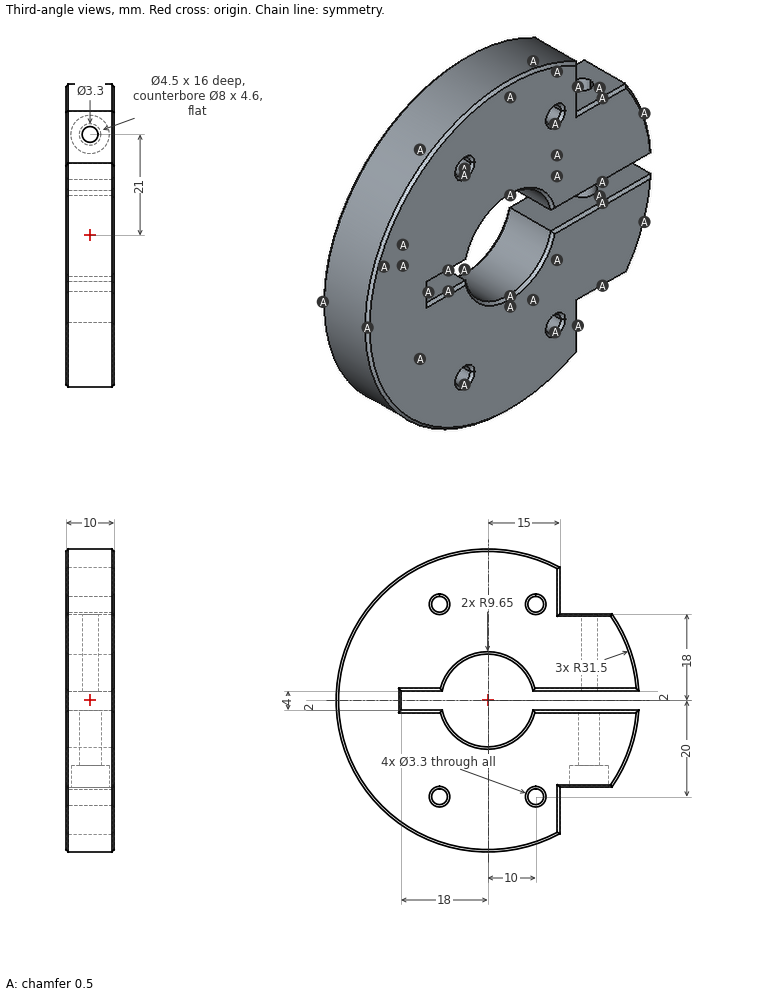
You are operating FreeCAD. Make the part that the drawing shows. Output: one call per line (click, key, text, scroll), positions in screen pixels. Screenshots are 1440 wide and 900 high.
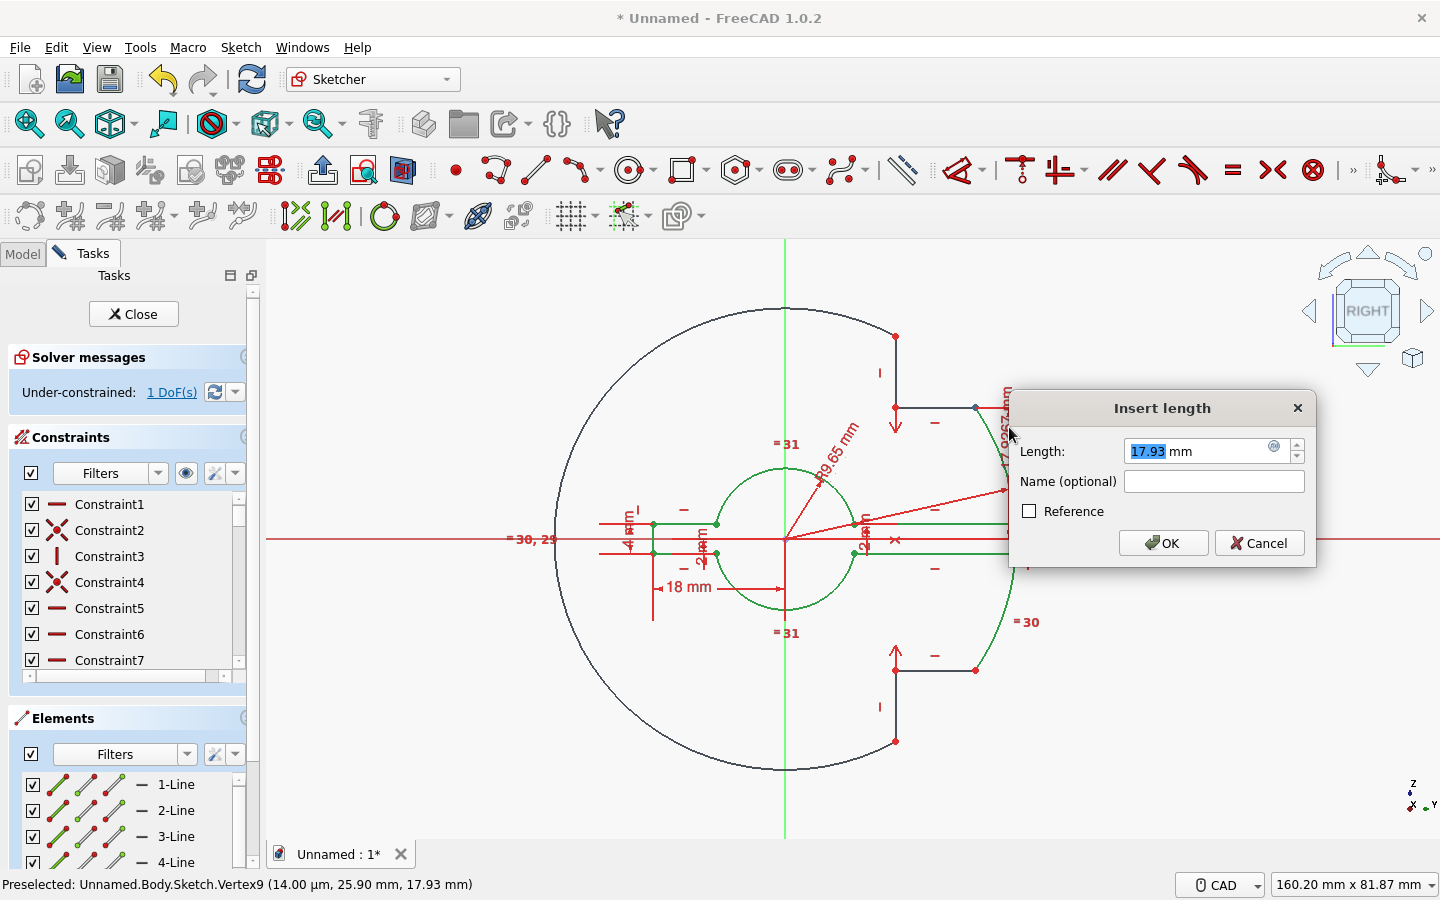
text(18)
key(Return)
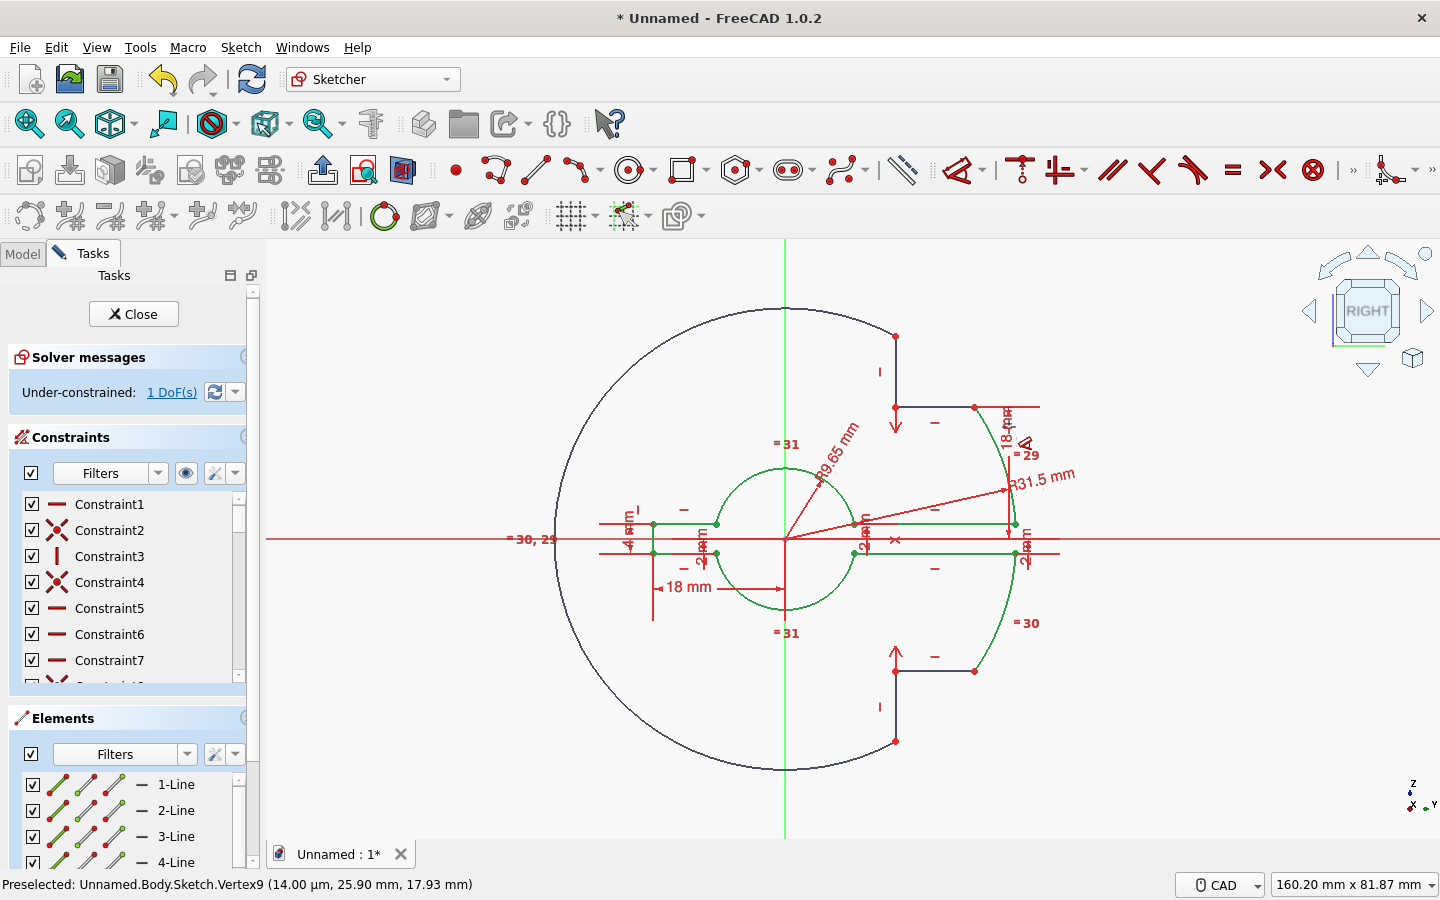
click(896, 407)
click(840, 373)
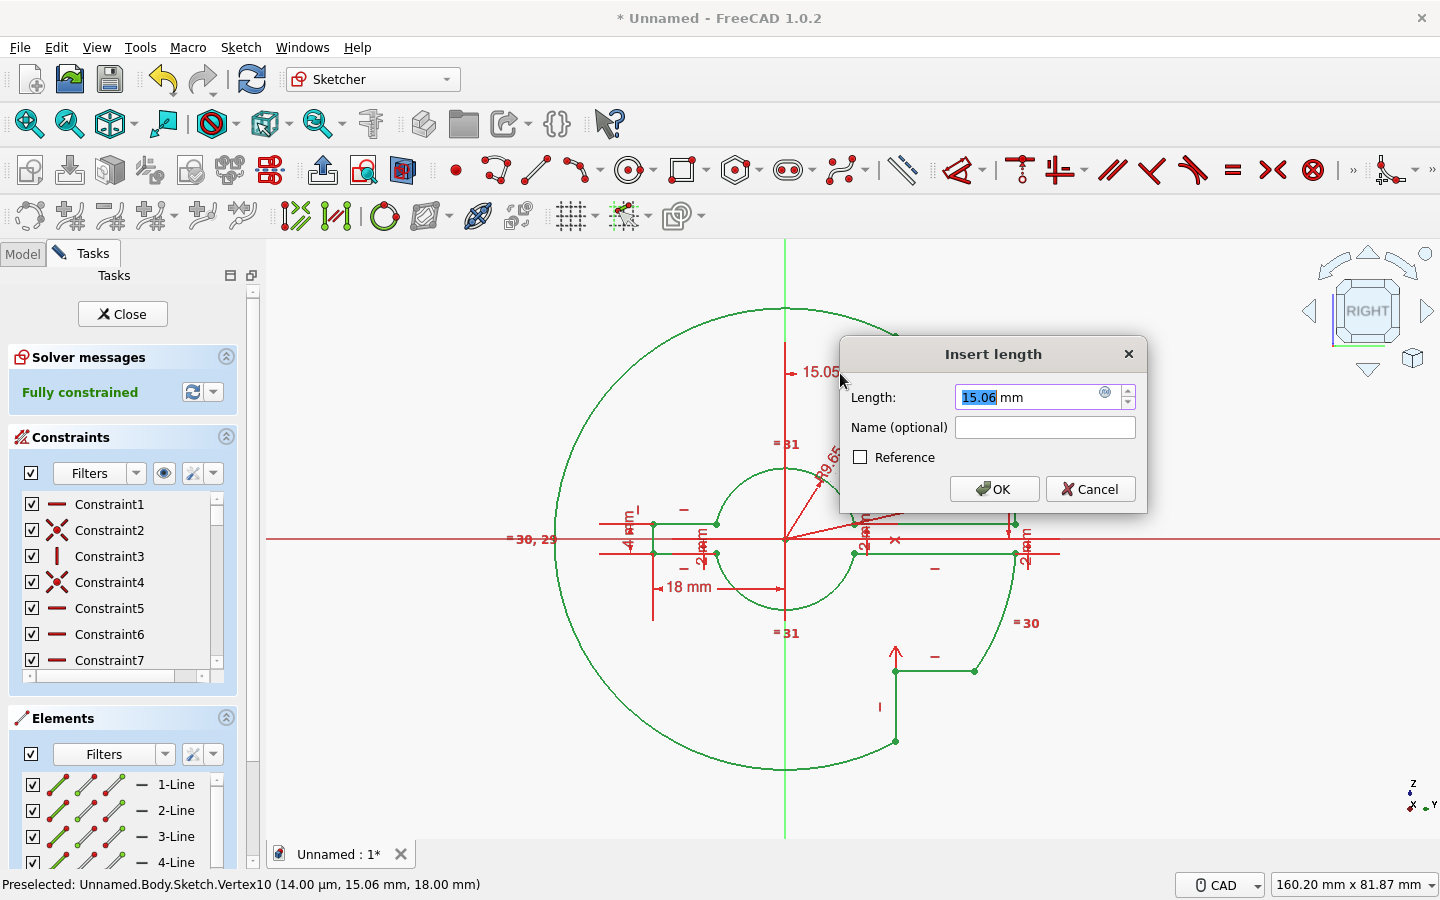
text(15)
key(Return)
key(Escape)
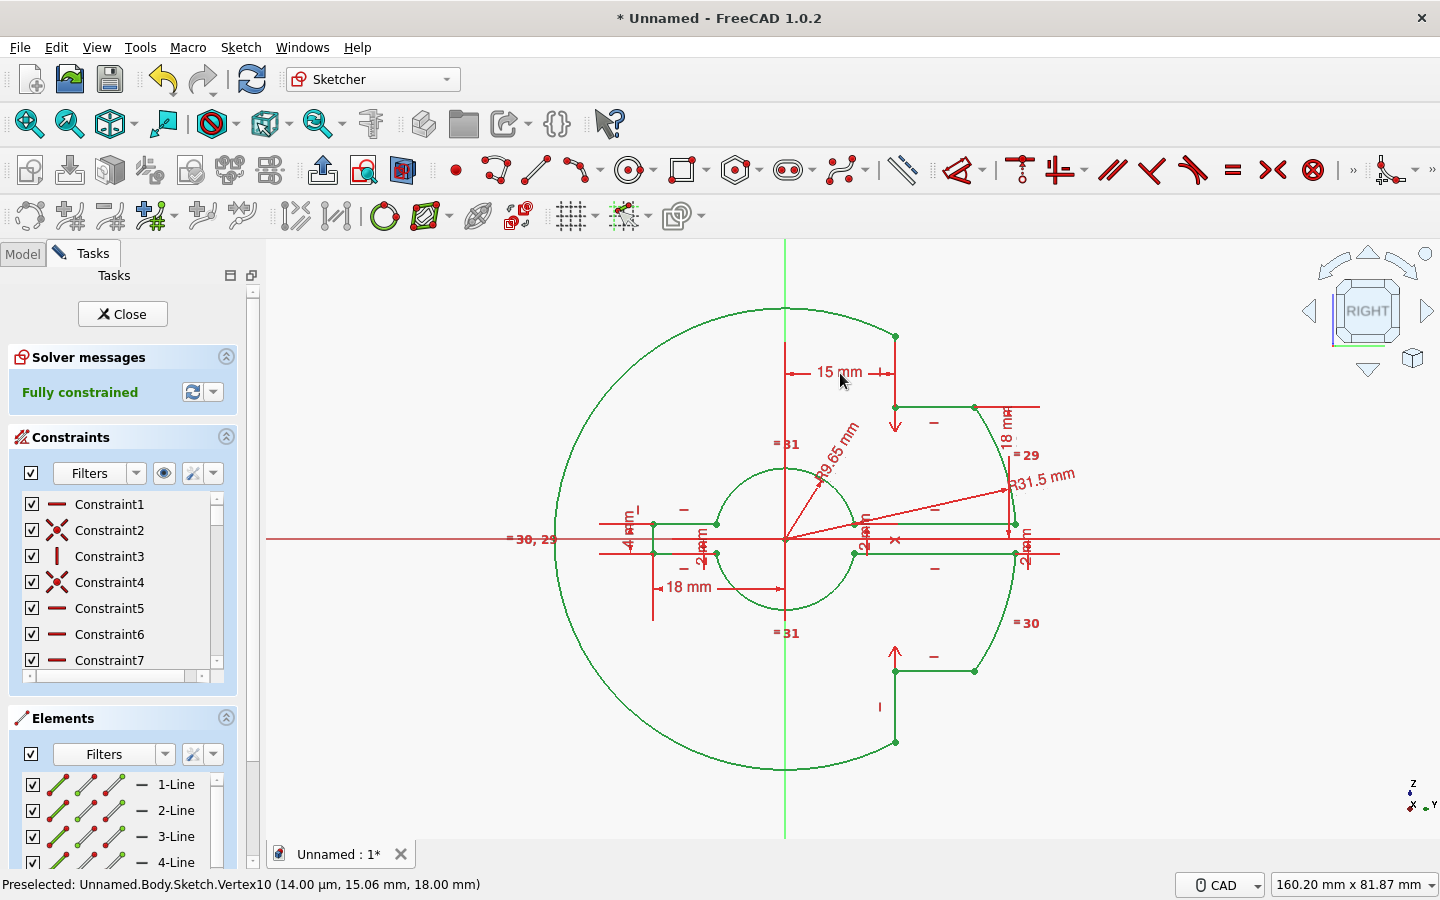
click(123, 314)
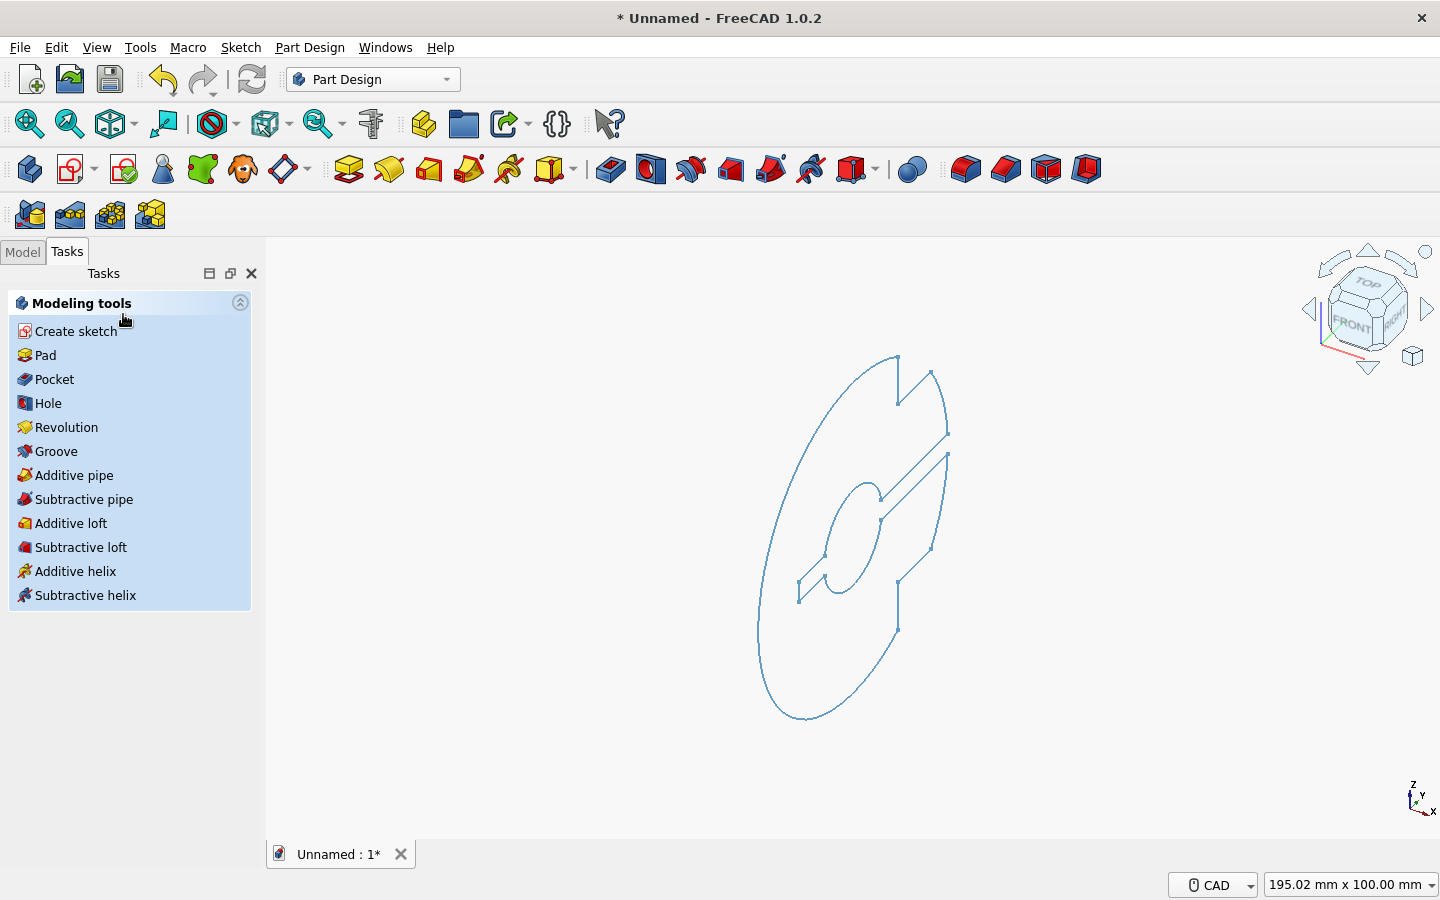
click(350, 170)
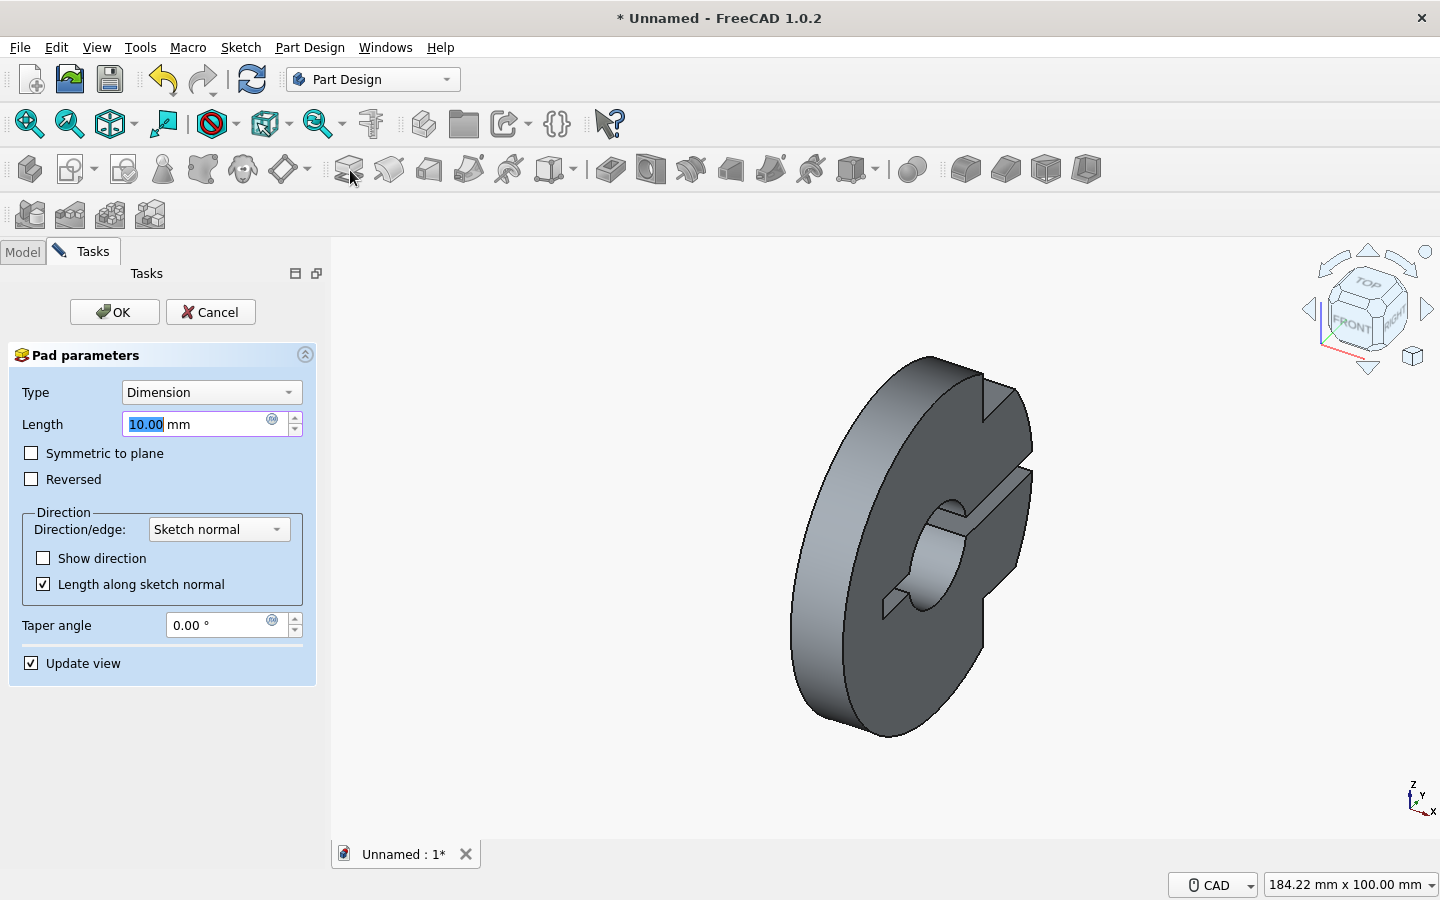
text(10)
key(Tab)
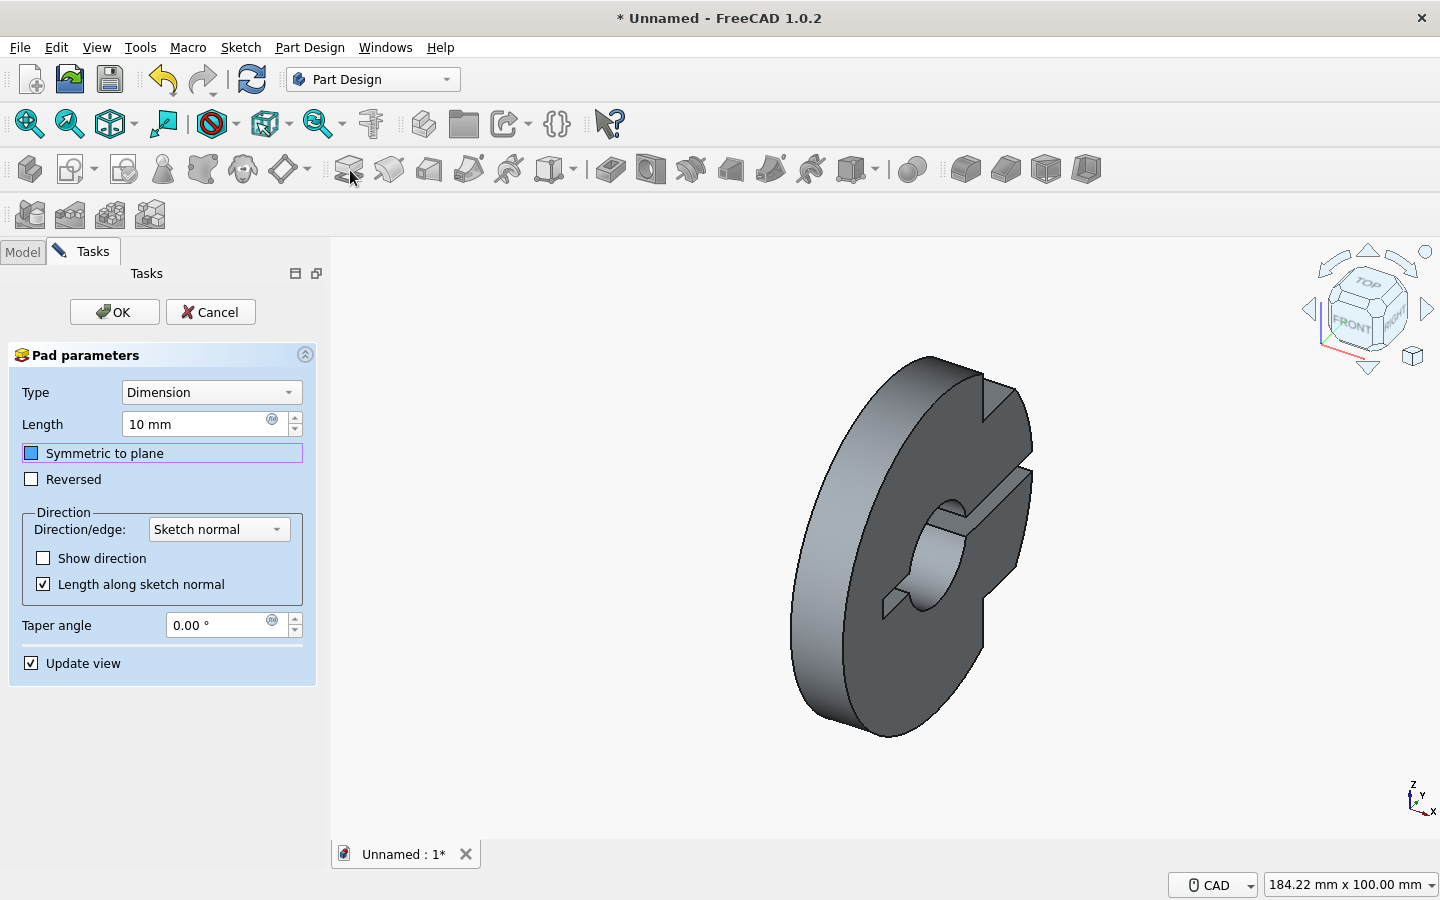
click(30, 453)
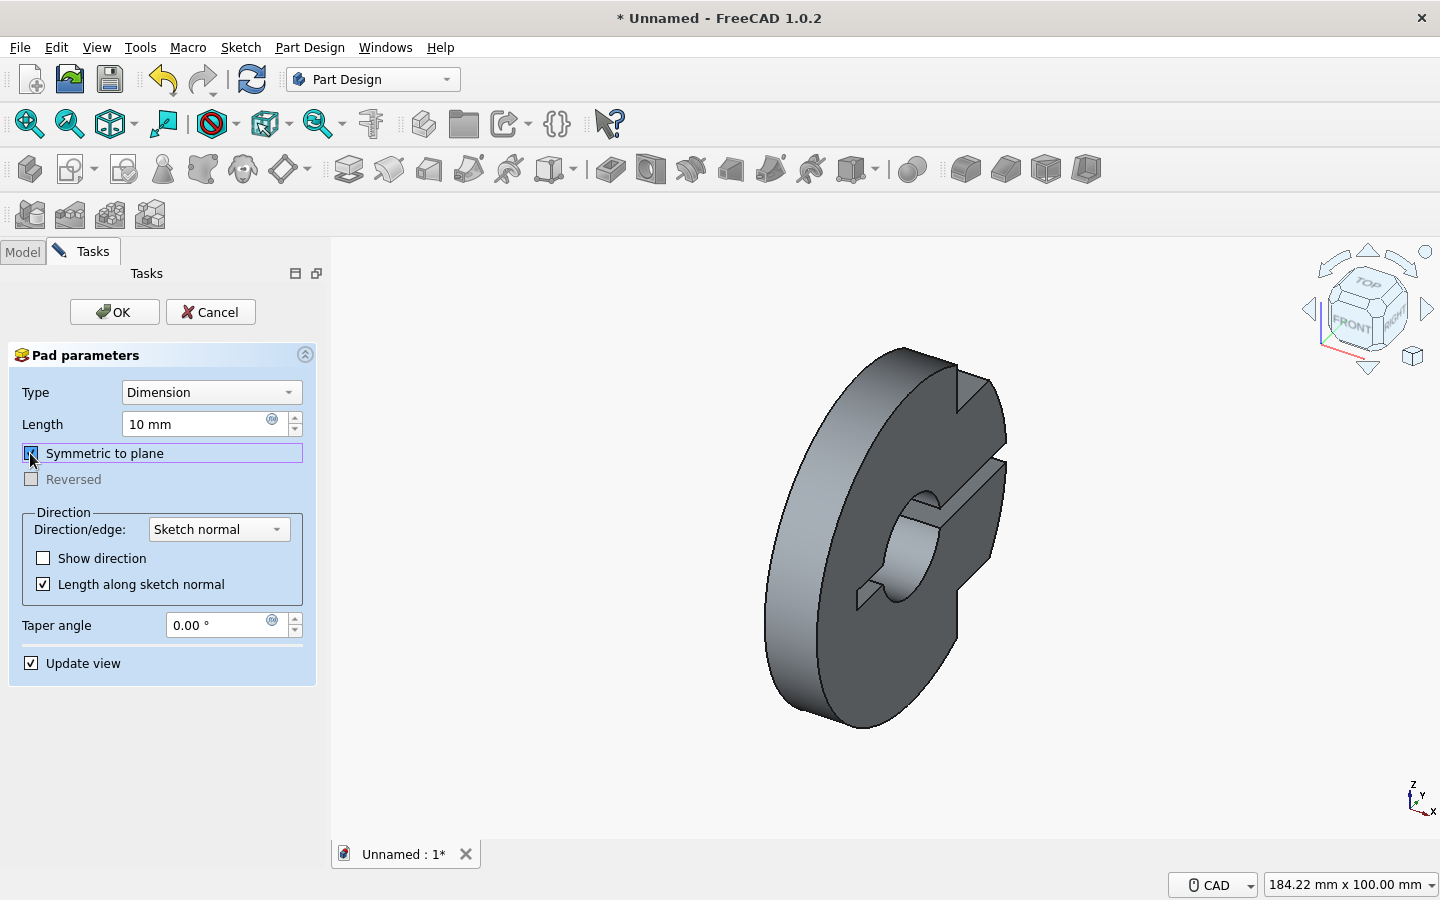
click(115, 312)